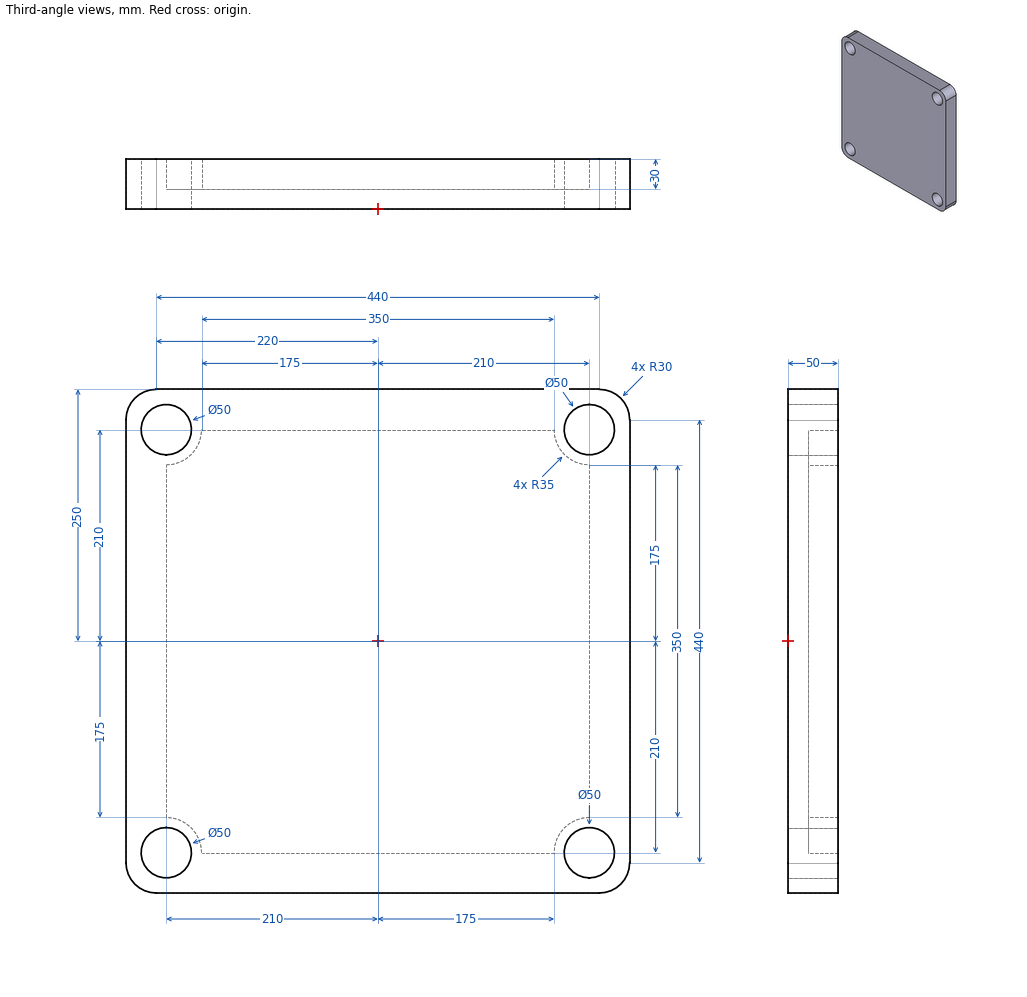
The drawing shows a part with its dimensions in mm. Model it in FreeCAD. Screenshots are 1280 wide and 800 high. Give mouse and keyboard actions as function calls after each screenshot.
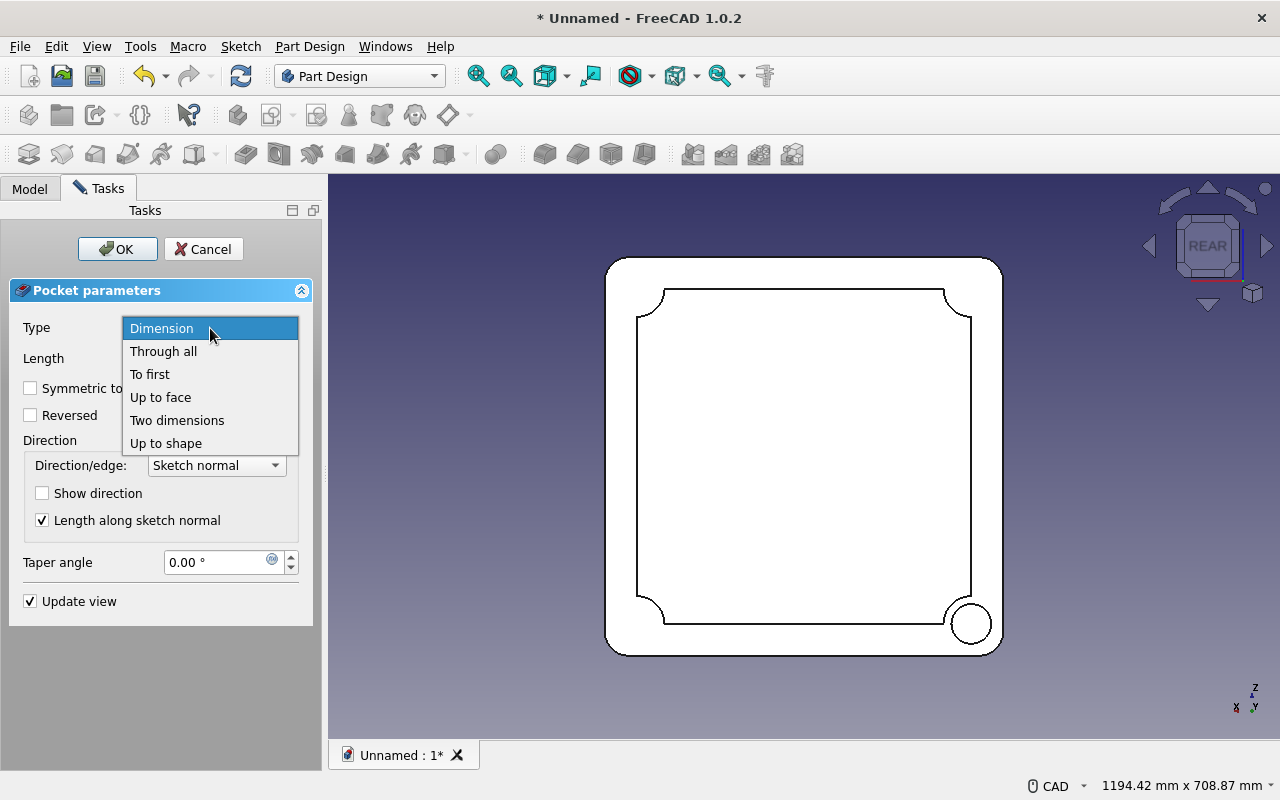
click(208, 374)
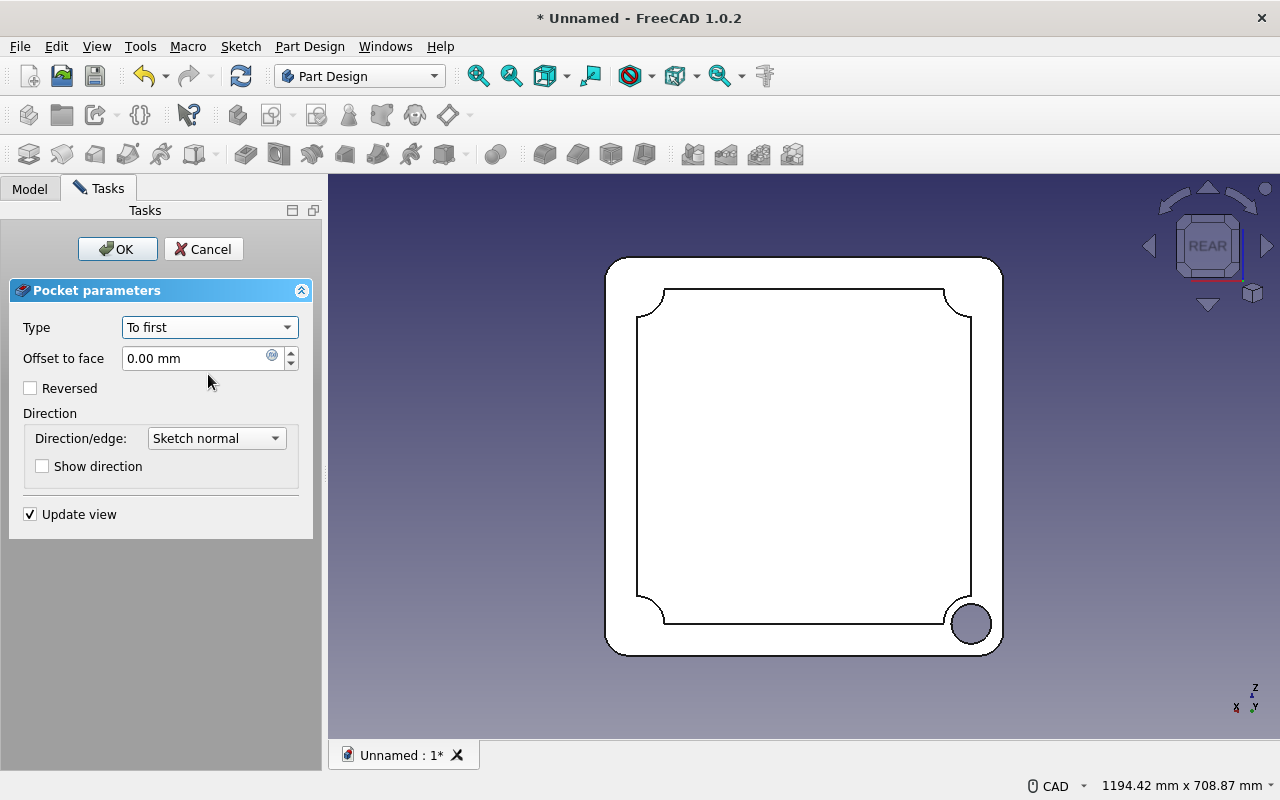
click(118, 249)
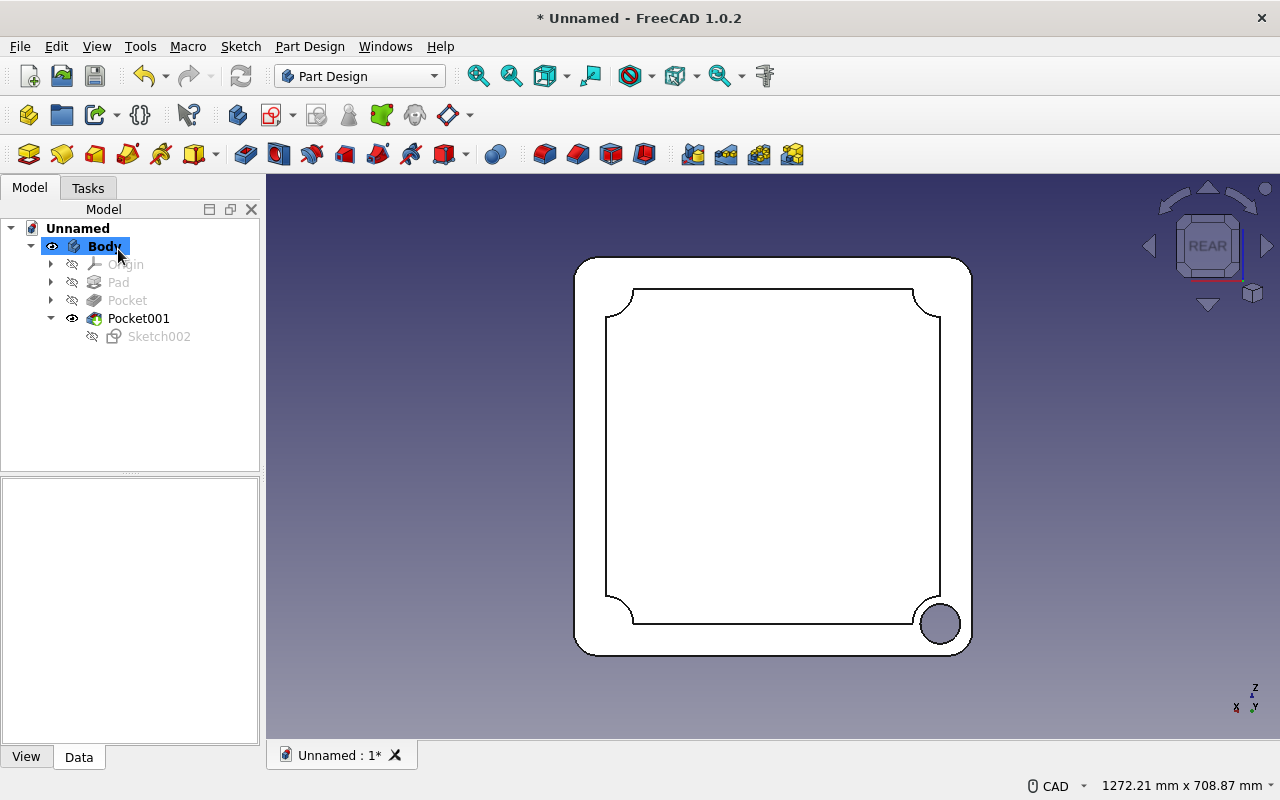
click(602, 285)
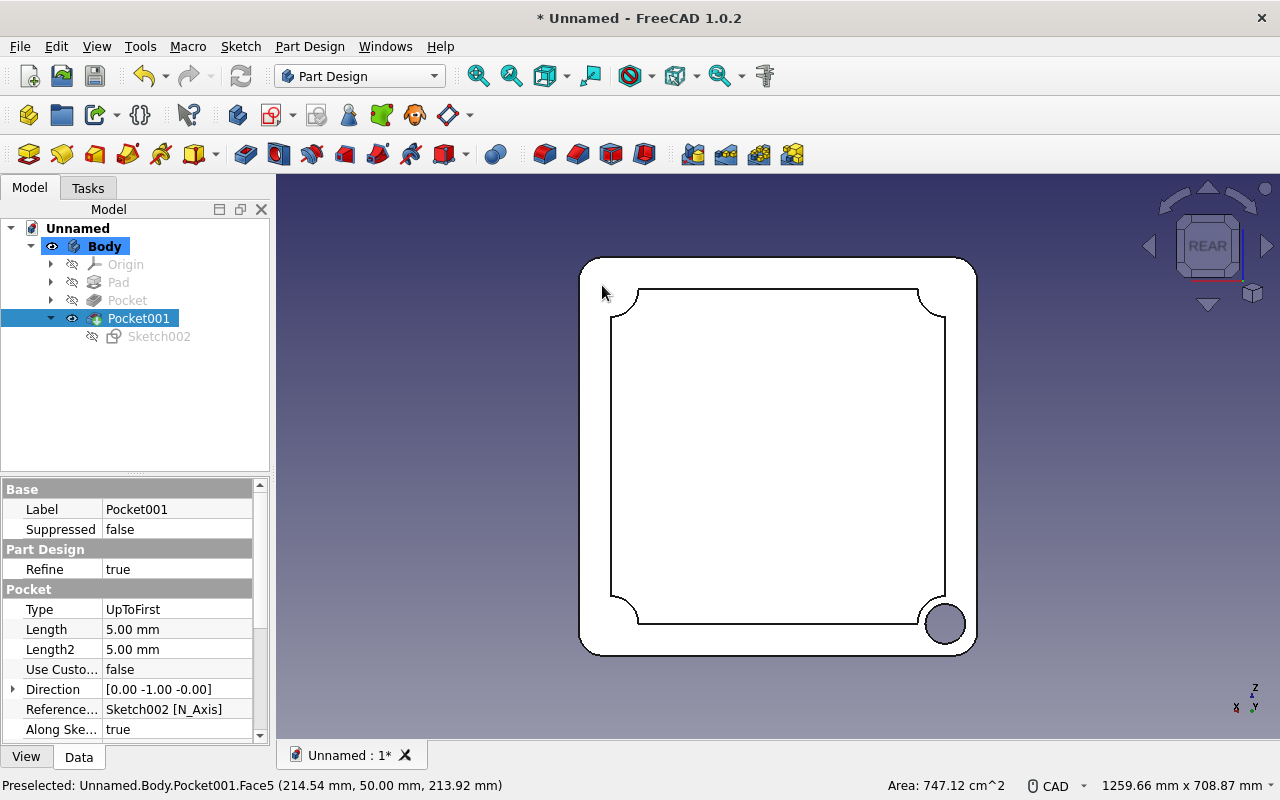
click(270, 116)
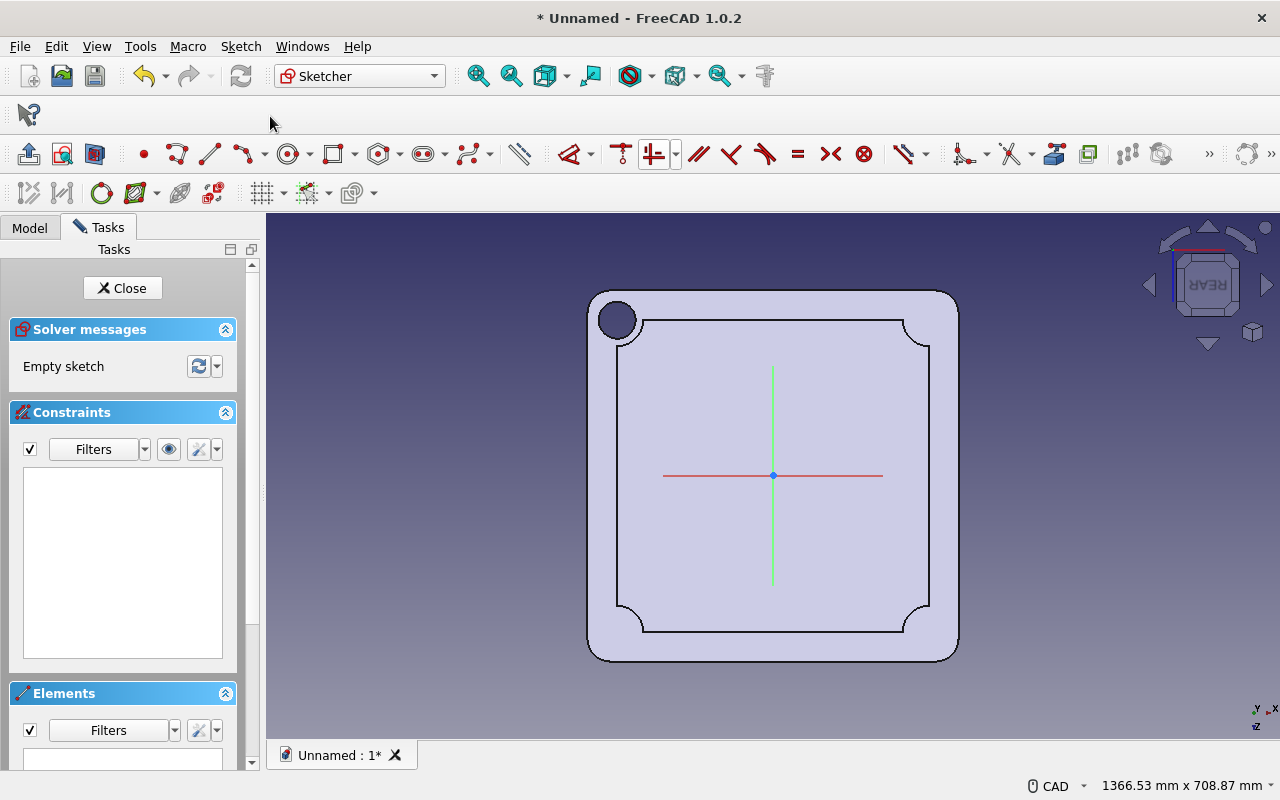
scroll(957, 301, up, 11)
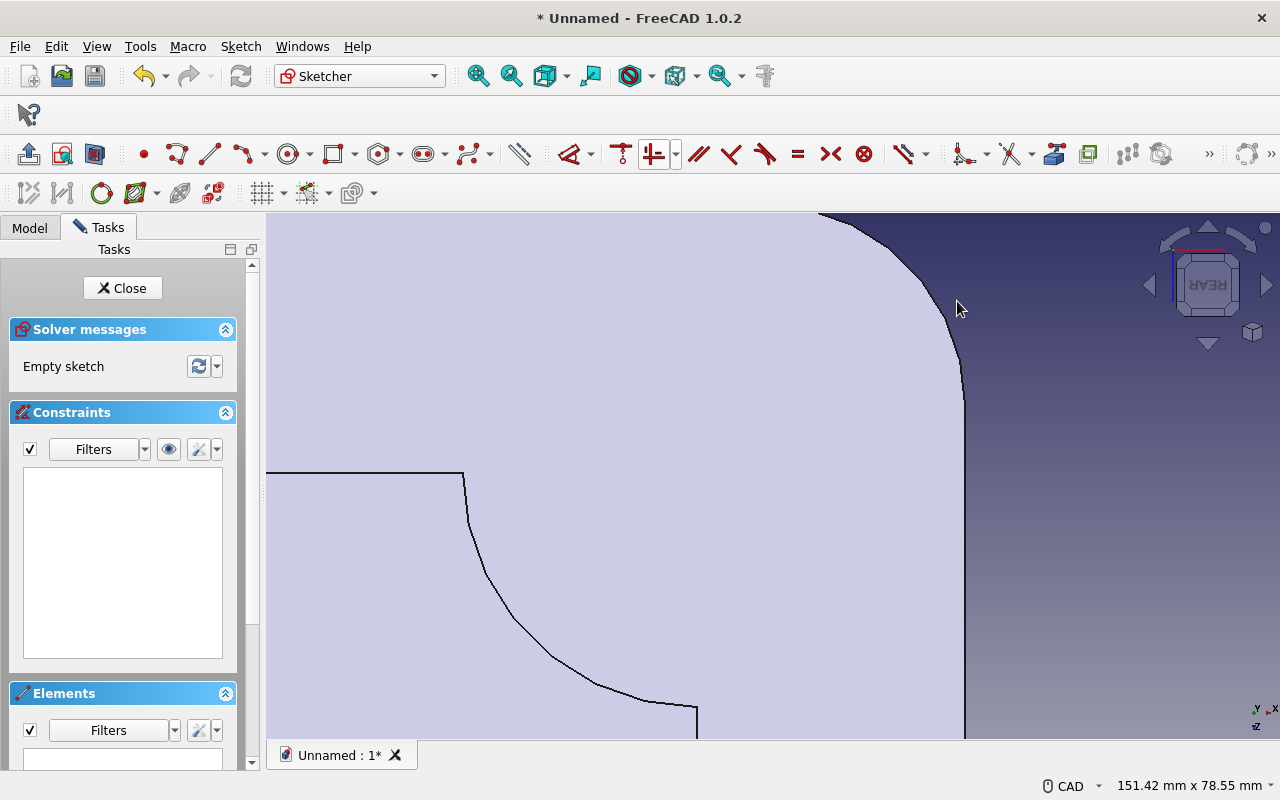
click(288, 154)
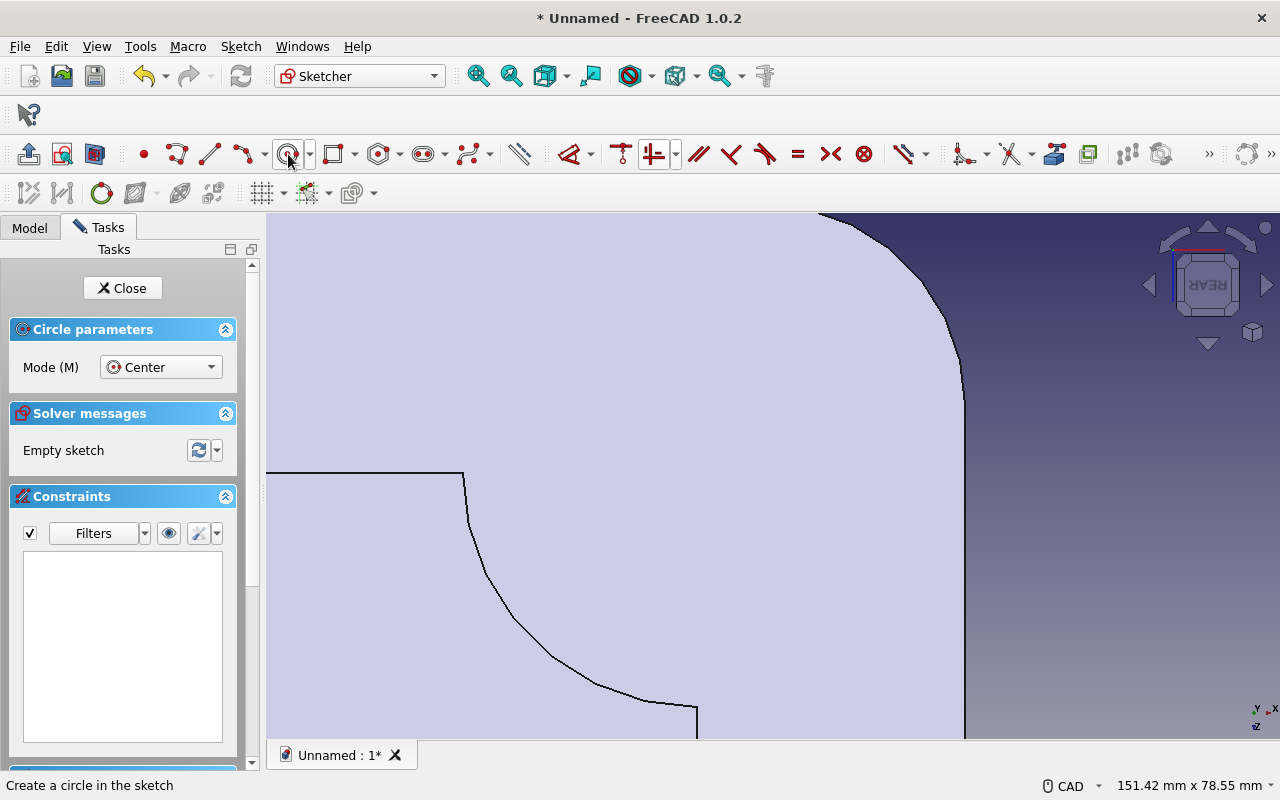
click(697, 473)
move(816, 354)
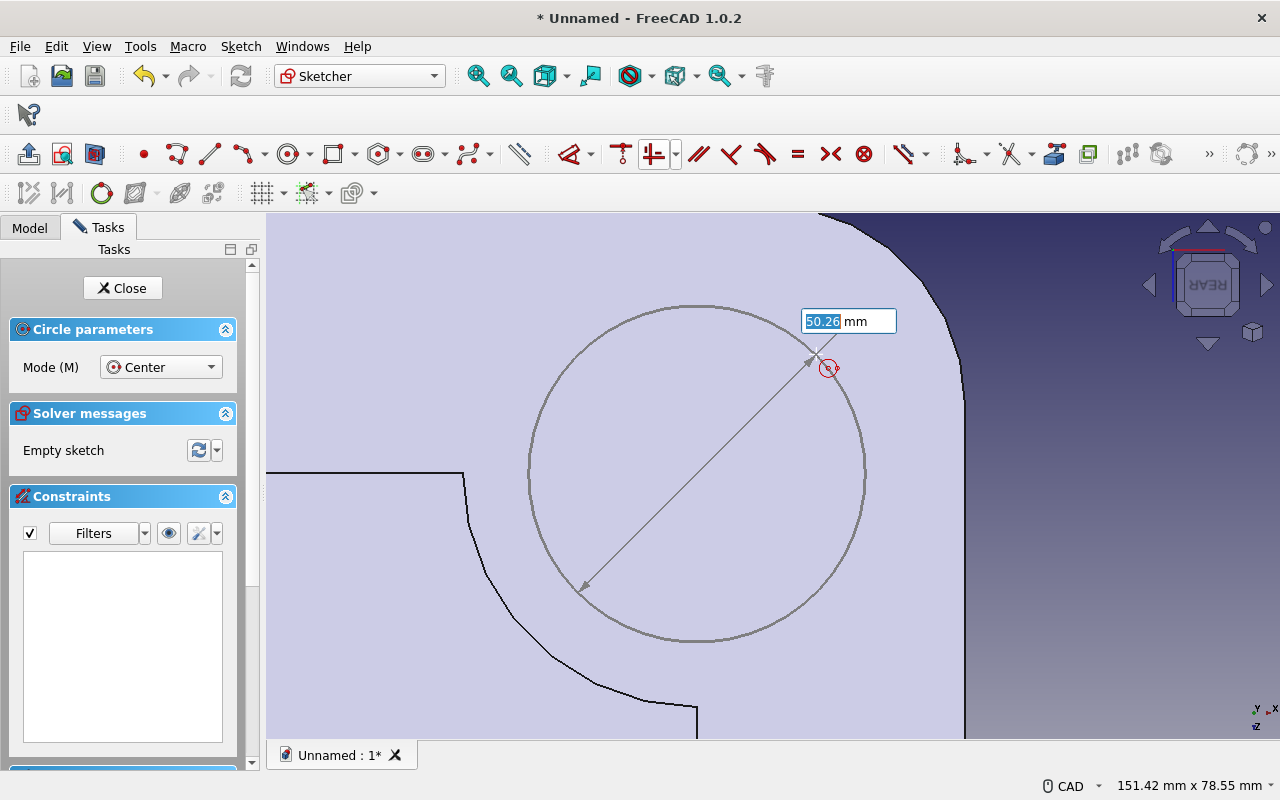
text(50)
key(Return)
key(Escape)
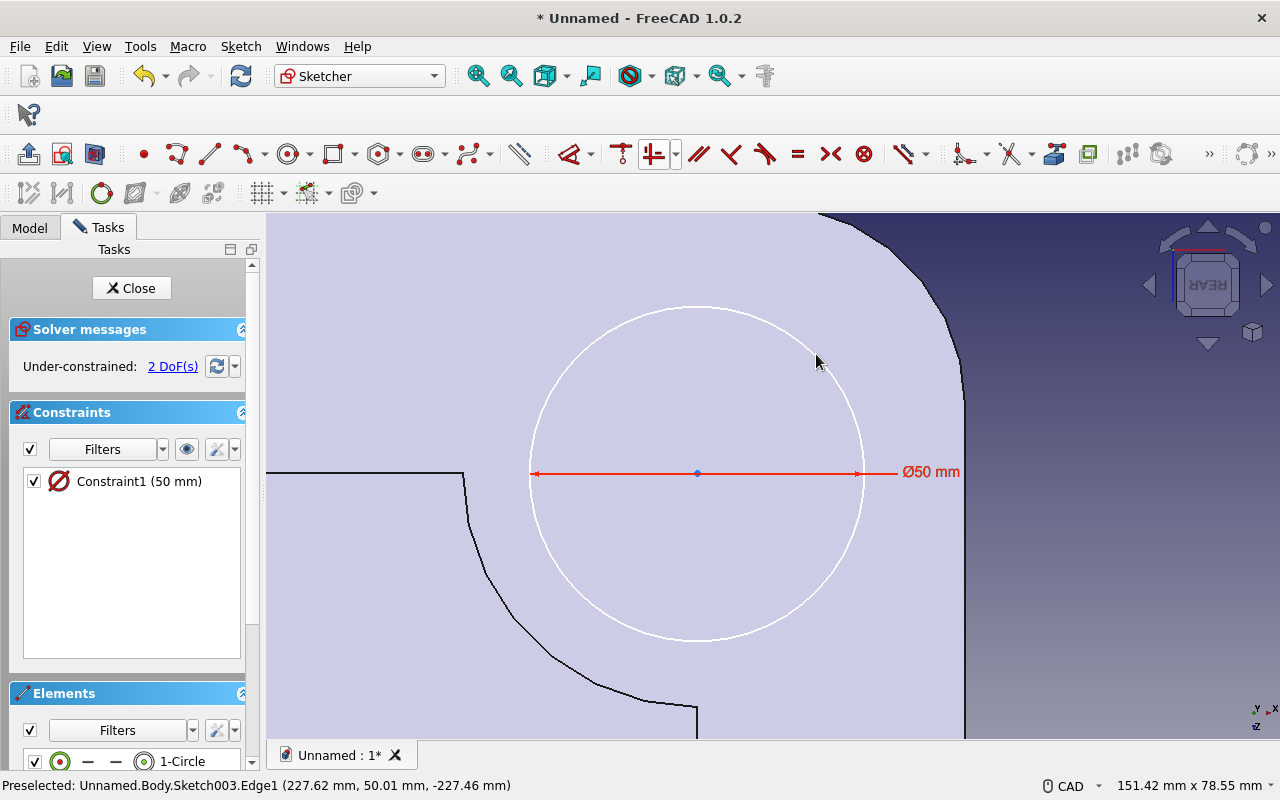
click(568, 154)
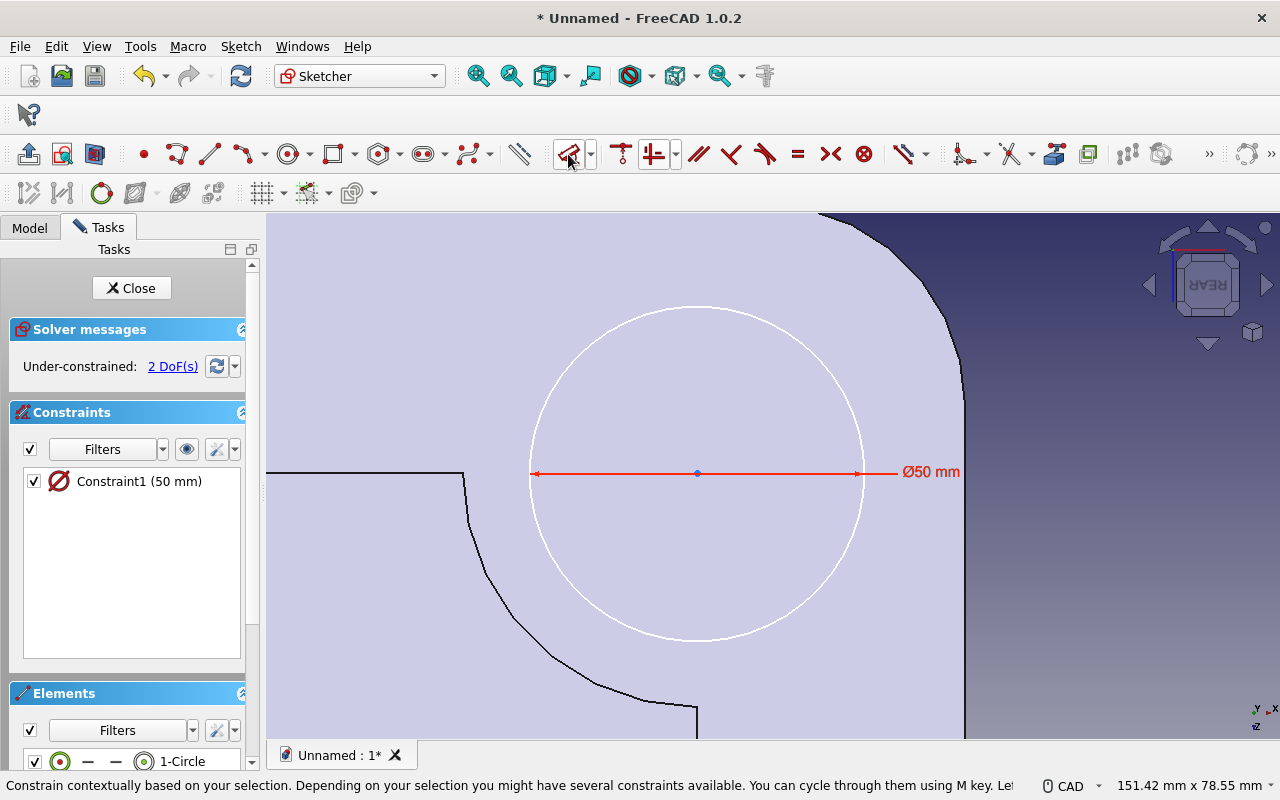
click(697, 474)
click(495, 440)